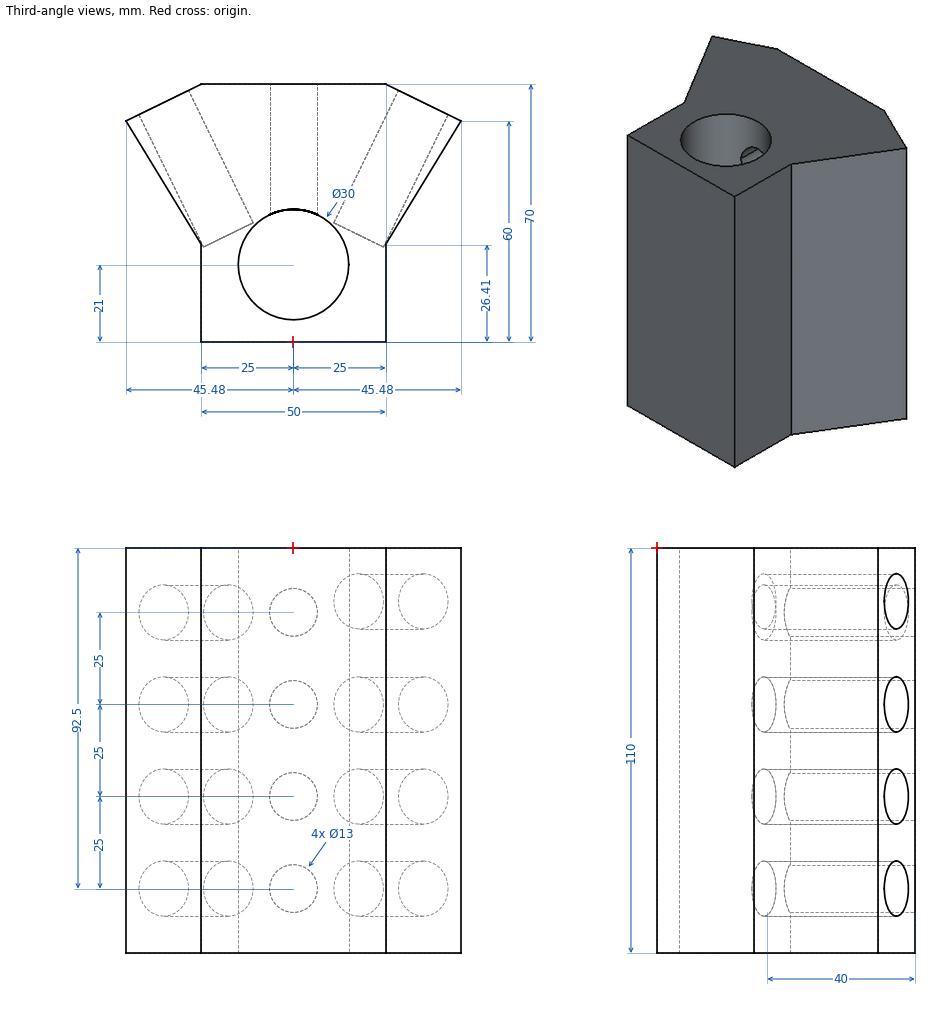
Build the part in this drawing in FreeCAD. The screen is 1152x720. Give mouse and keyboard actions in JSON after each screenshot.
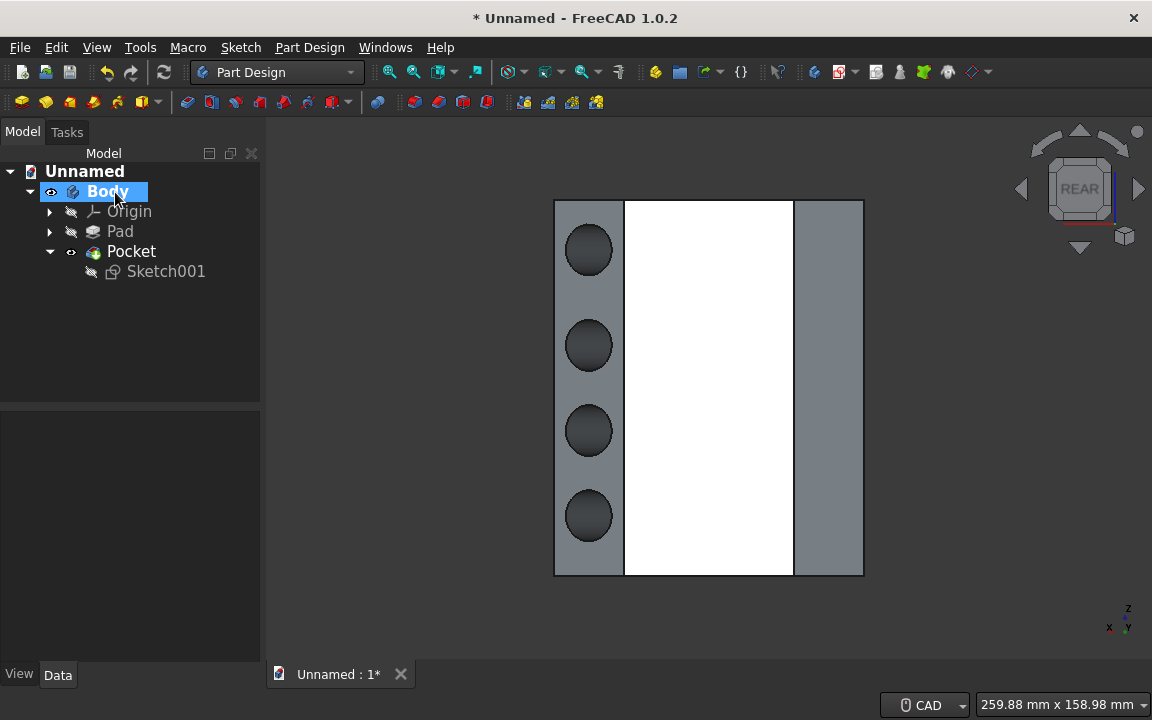
{"action": "left_click", "coordinate": [829, 280]}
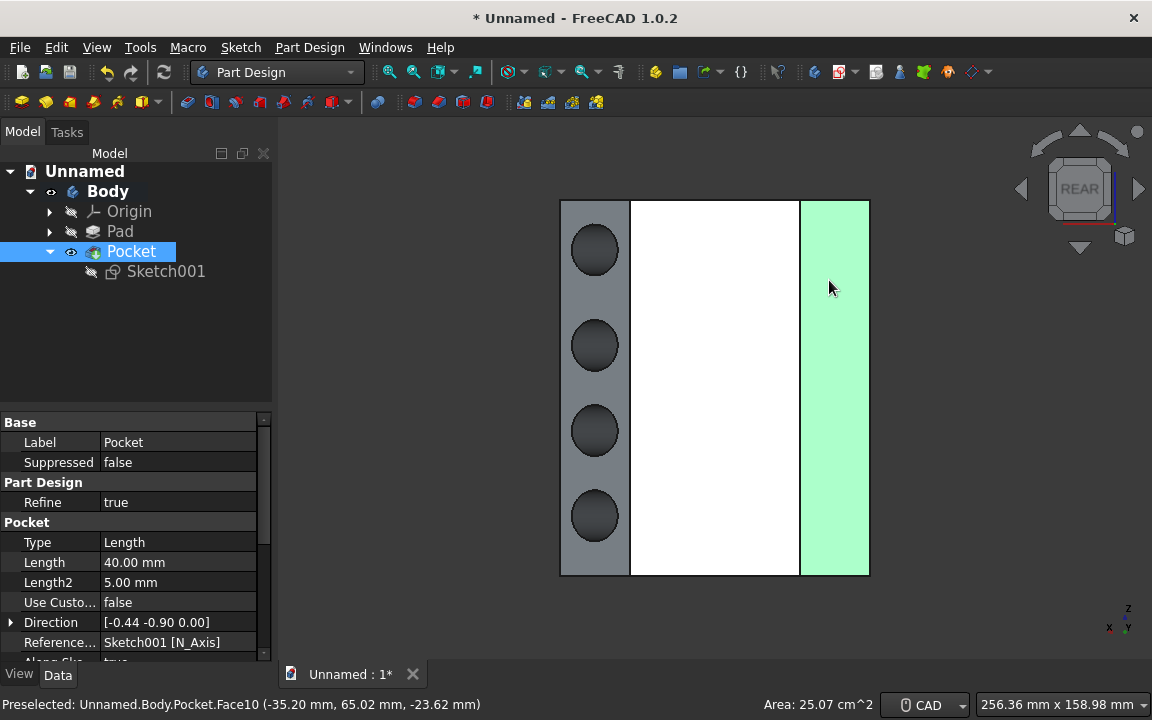
{"action": "left_click", "coordinate": [840, 72]}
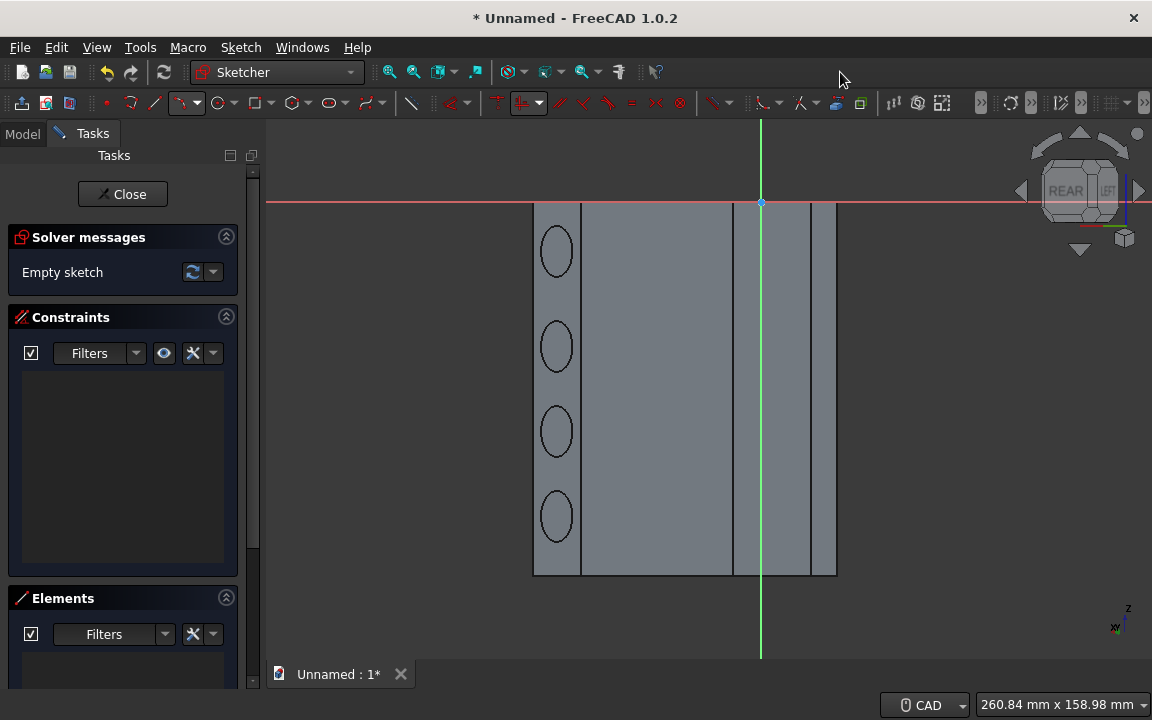
{"action": "key", "text": "q s"}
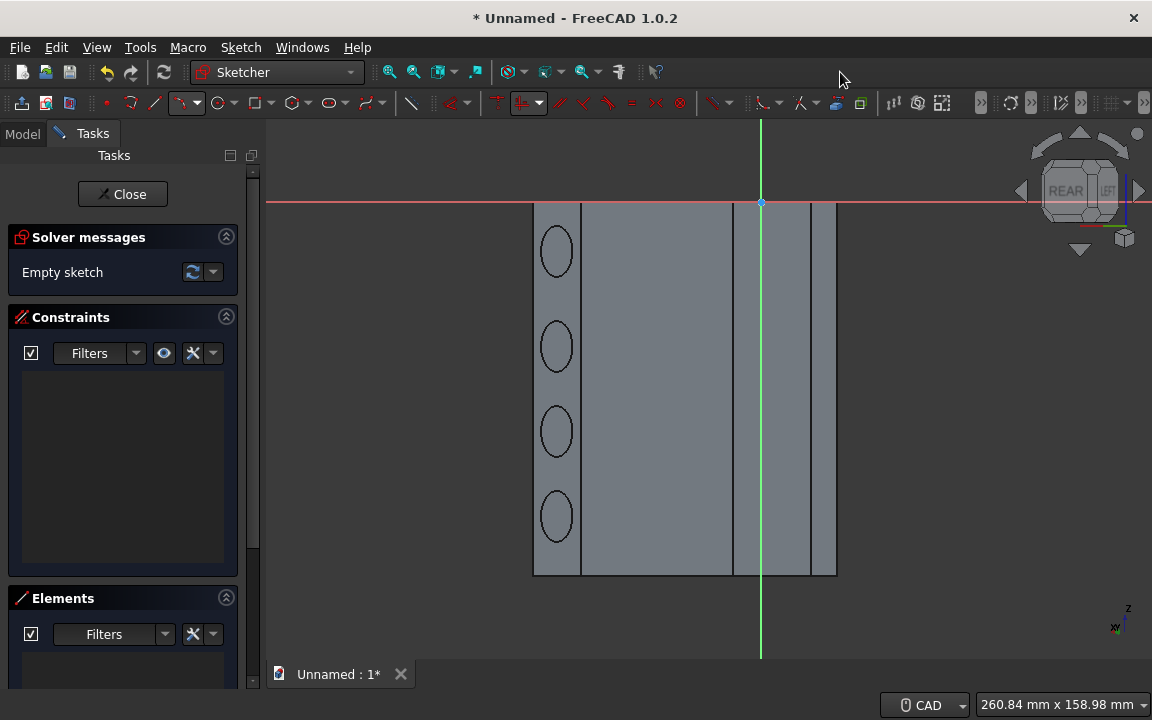
{"action": "key", "text": "g c"}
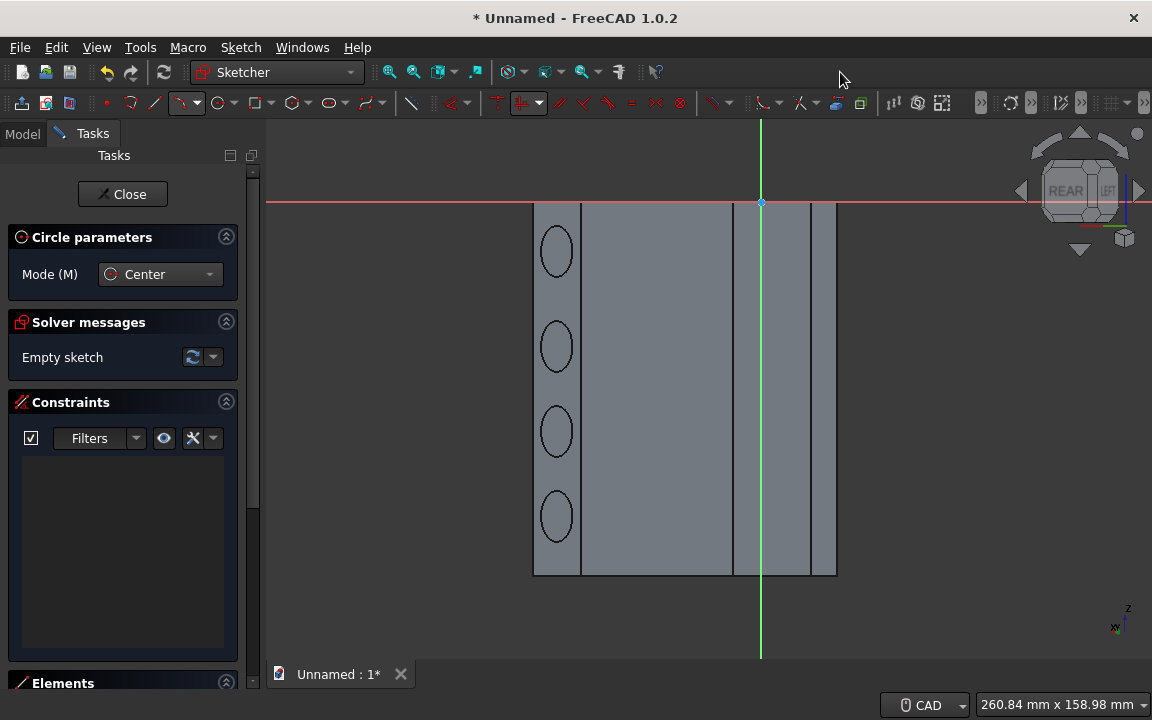
{"action": "scroll", "coordinate": [772, 516], "scroll_direction": "up", "scroll_amount": 2}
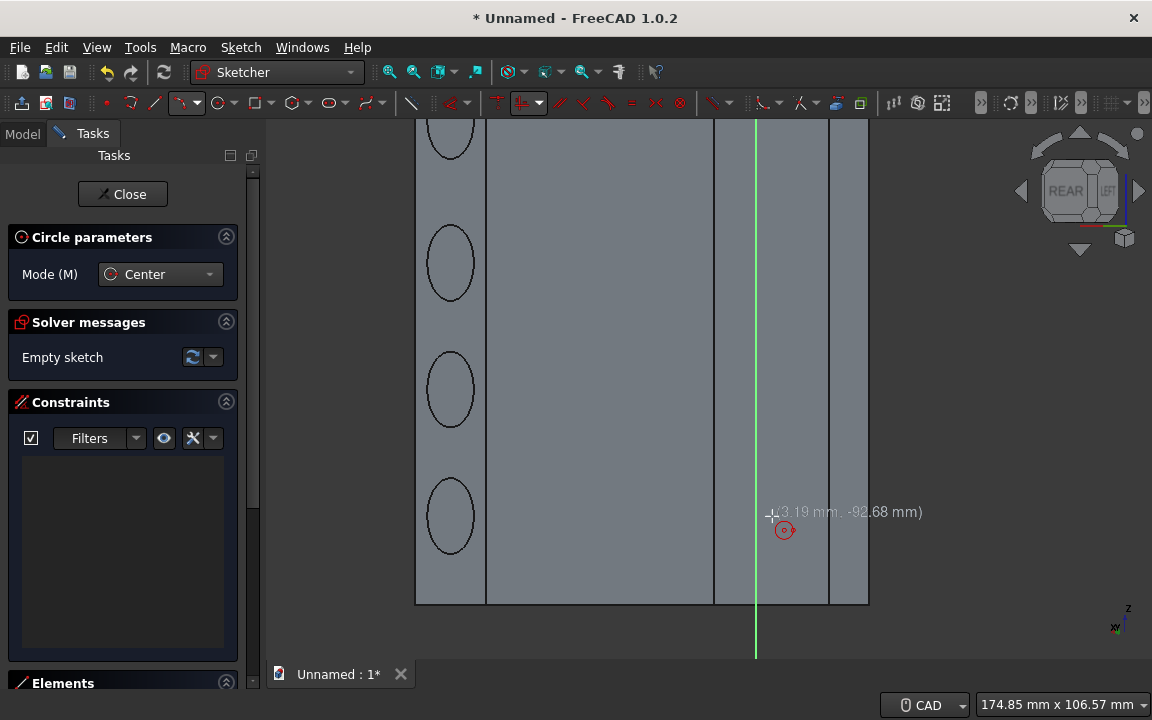
{"action": "left_click", "coordinate": [771, 516]}
{"action": "left_click", "coordinate": [798, 489]}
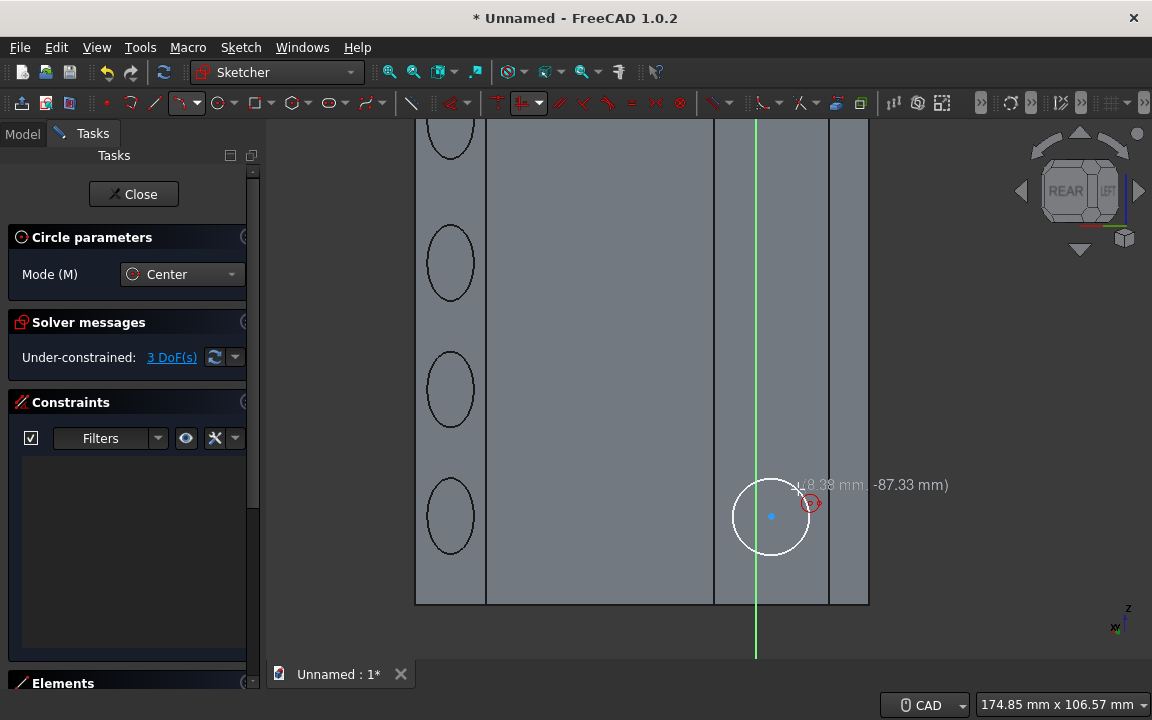
{"action": "left_click", "coordinate": [771, 390]}
{"action": "left_click", "coordinate": [798, 363]}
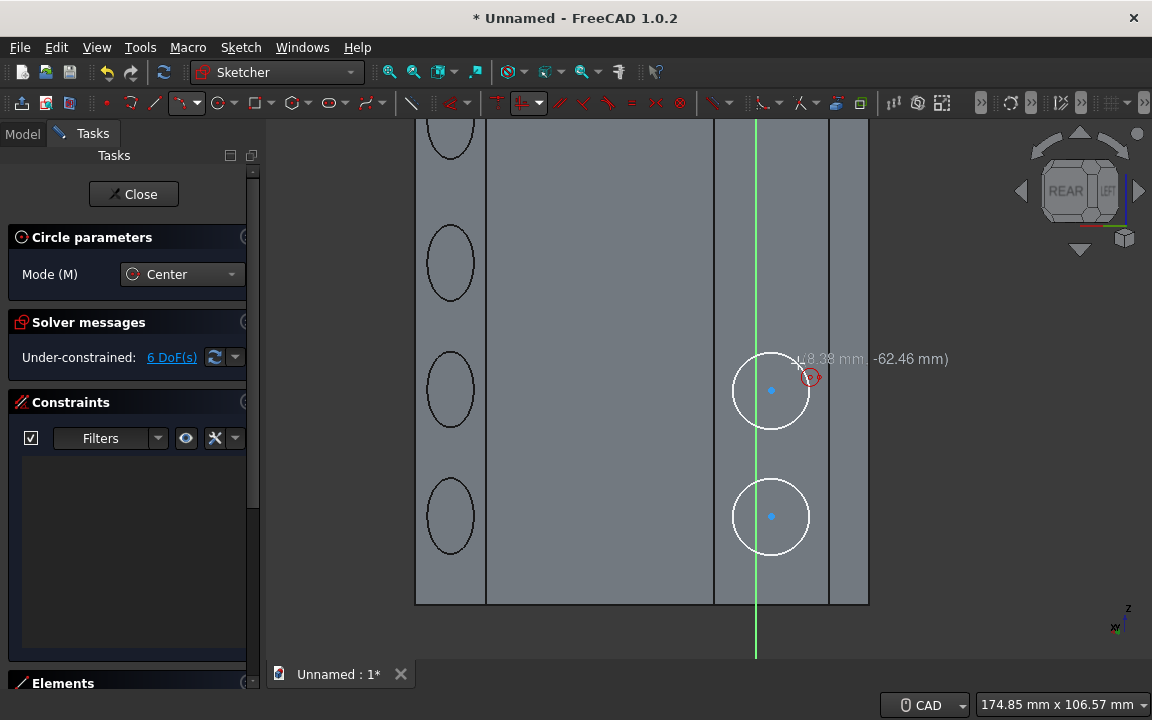
{"action": "left_click", "coordinate": [771, 263]}
{"action": "left_click", "coordinate": [798, 236]}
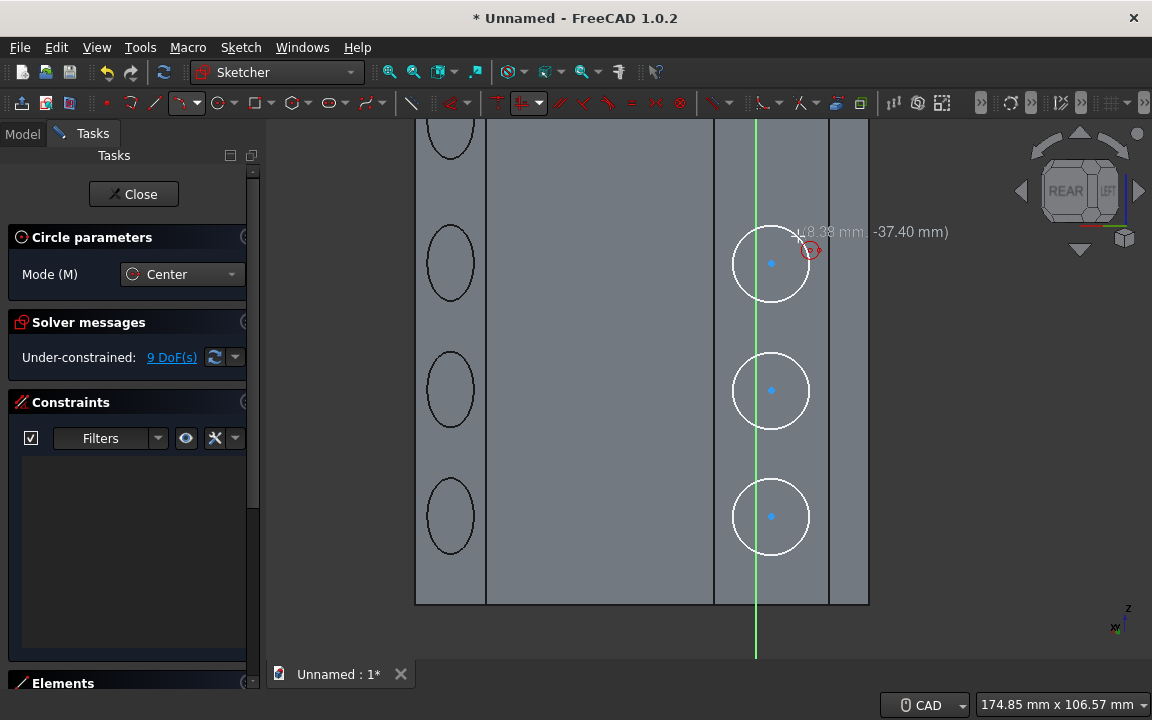
{"action": "scroll", "coordinate": [374, 568], "scroll_direction": "down", "scroll_amount": 2}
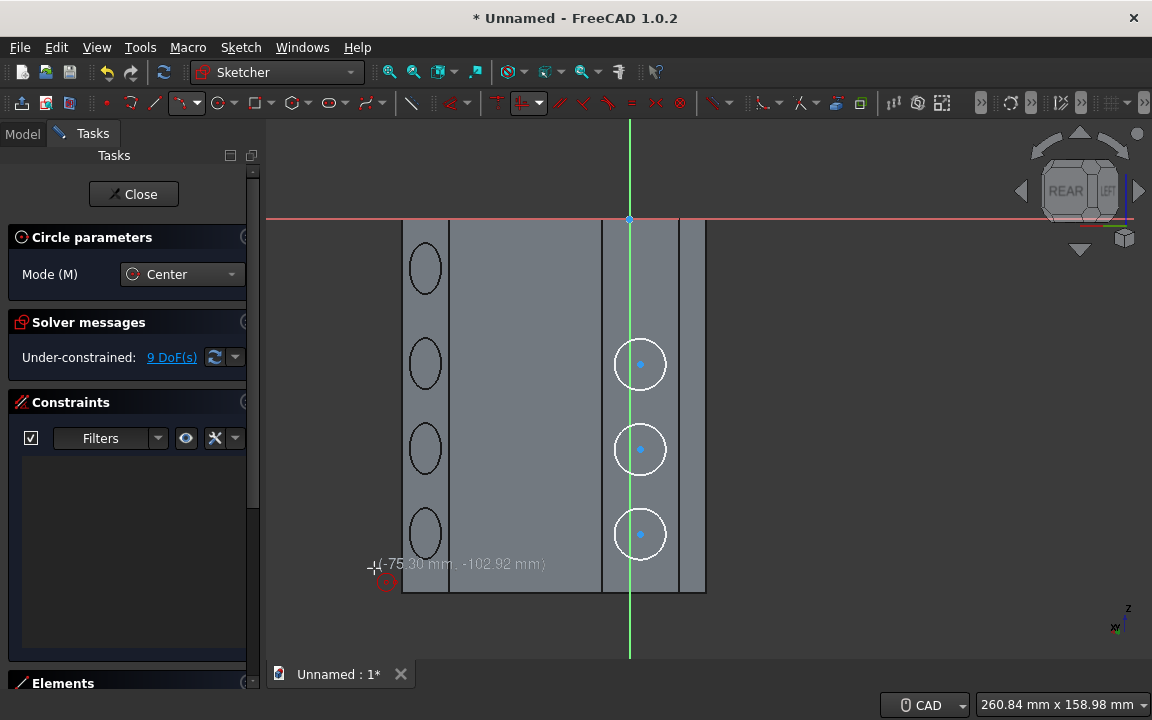
{"action": "scroll", "coordinate": [640, 279], "scroll_direction": "up", "scroll_amount": 2}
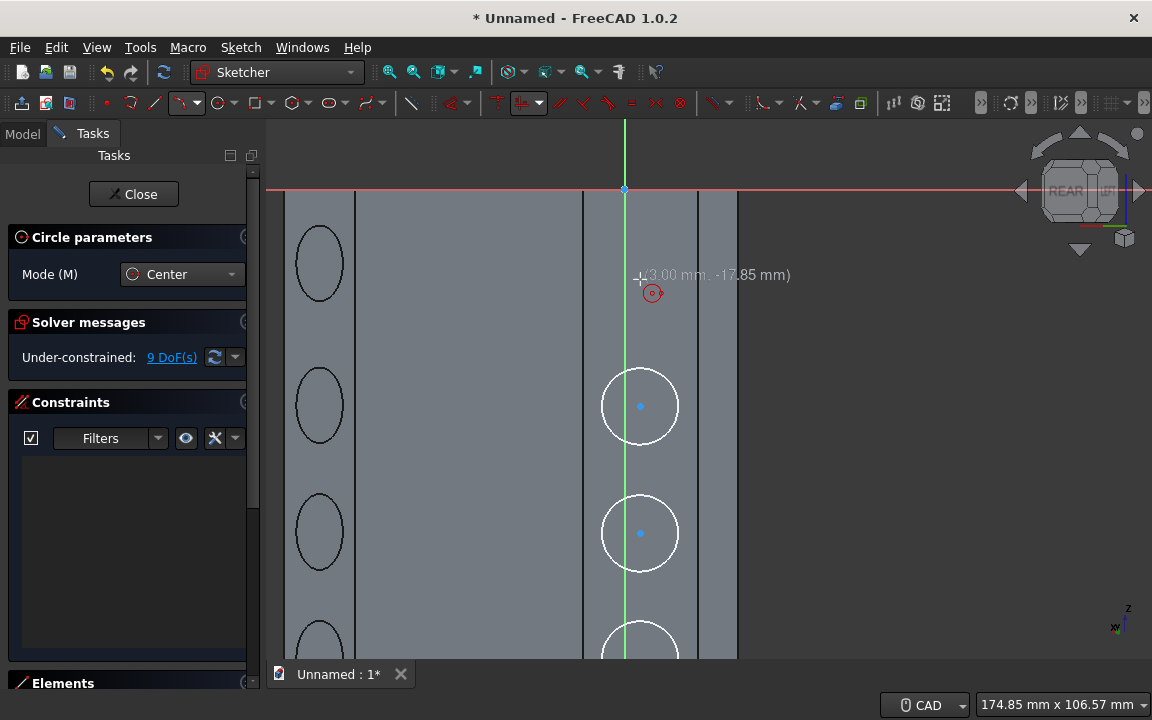
{"action": "left_click", "coordinate": [641, 279]}
{"action": "left_click", "coordinate": [667, 252]}
{"action": "key", "text": "Escape"}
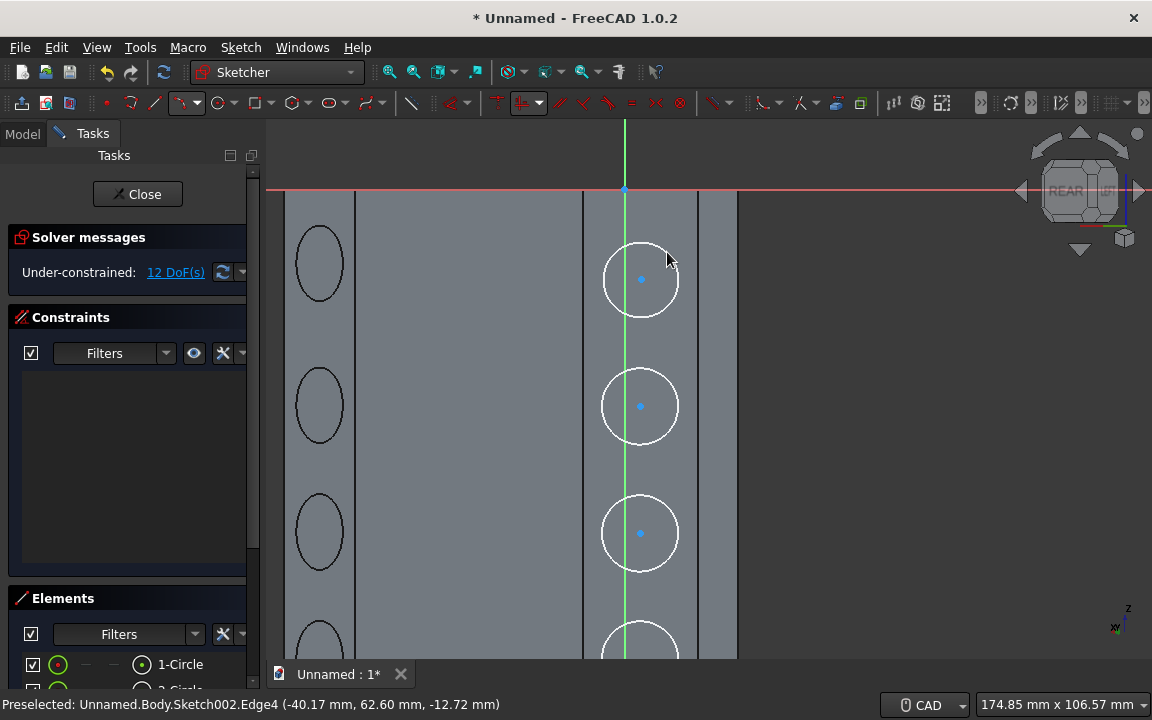
{"action": "left_click", "coordinate": [641, 621]}